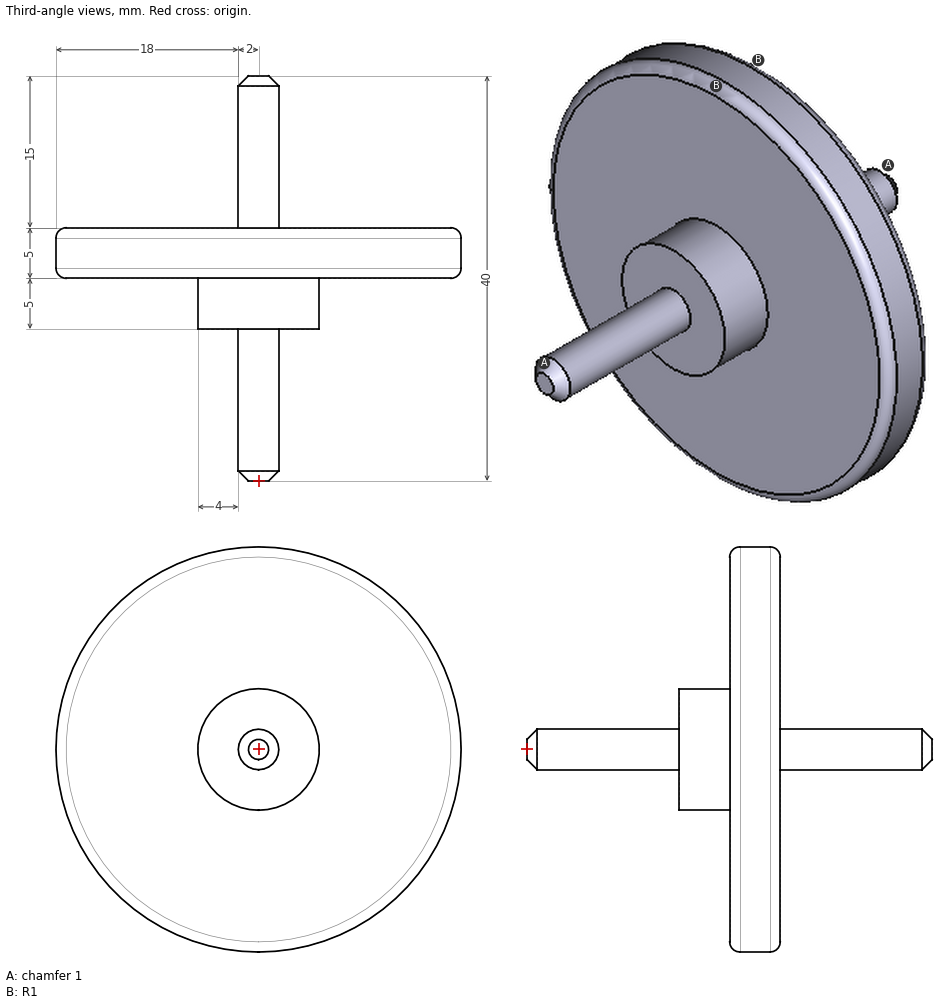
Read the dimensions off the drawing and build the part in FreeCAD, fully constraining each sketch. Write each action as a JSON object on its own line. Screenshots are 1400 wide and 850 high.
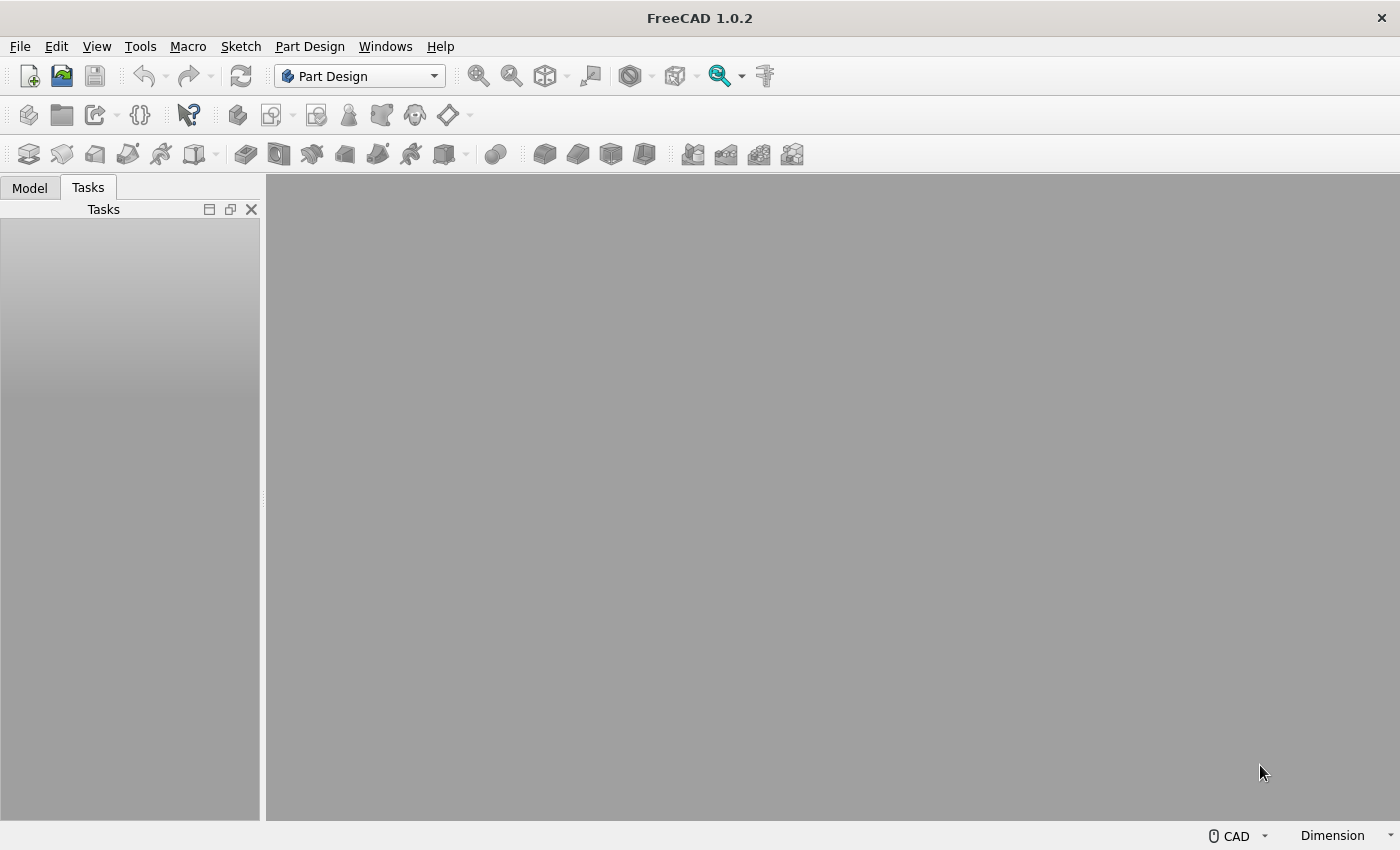
{"action": "key", "text": "ctrl+n"}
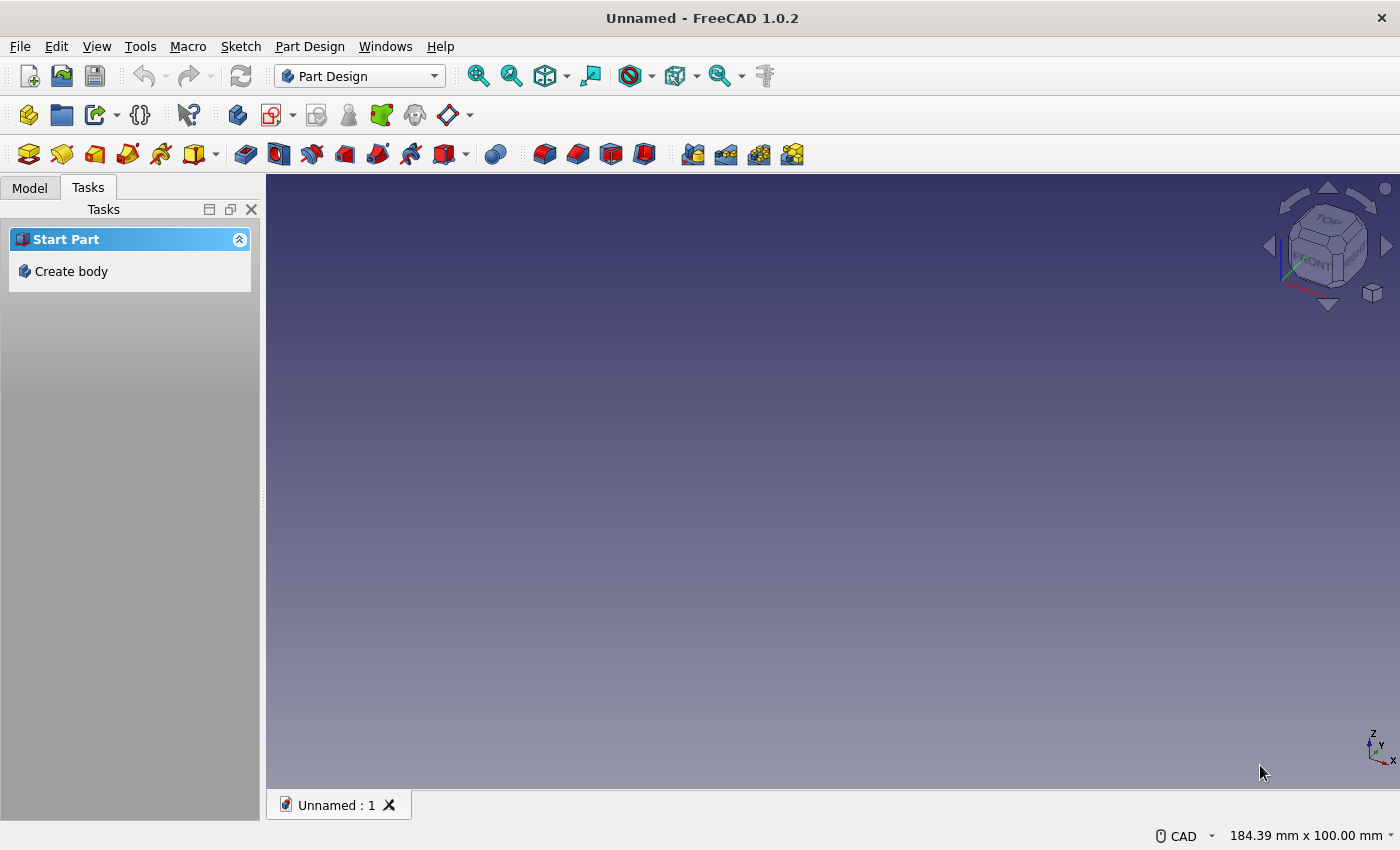
{"action": "left_click", "coordinate": [270, 116]}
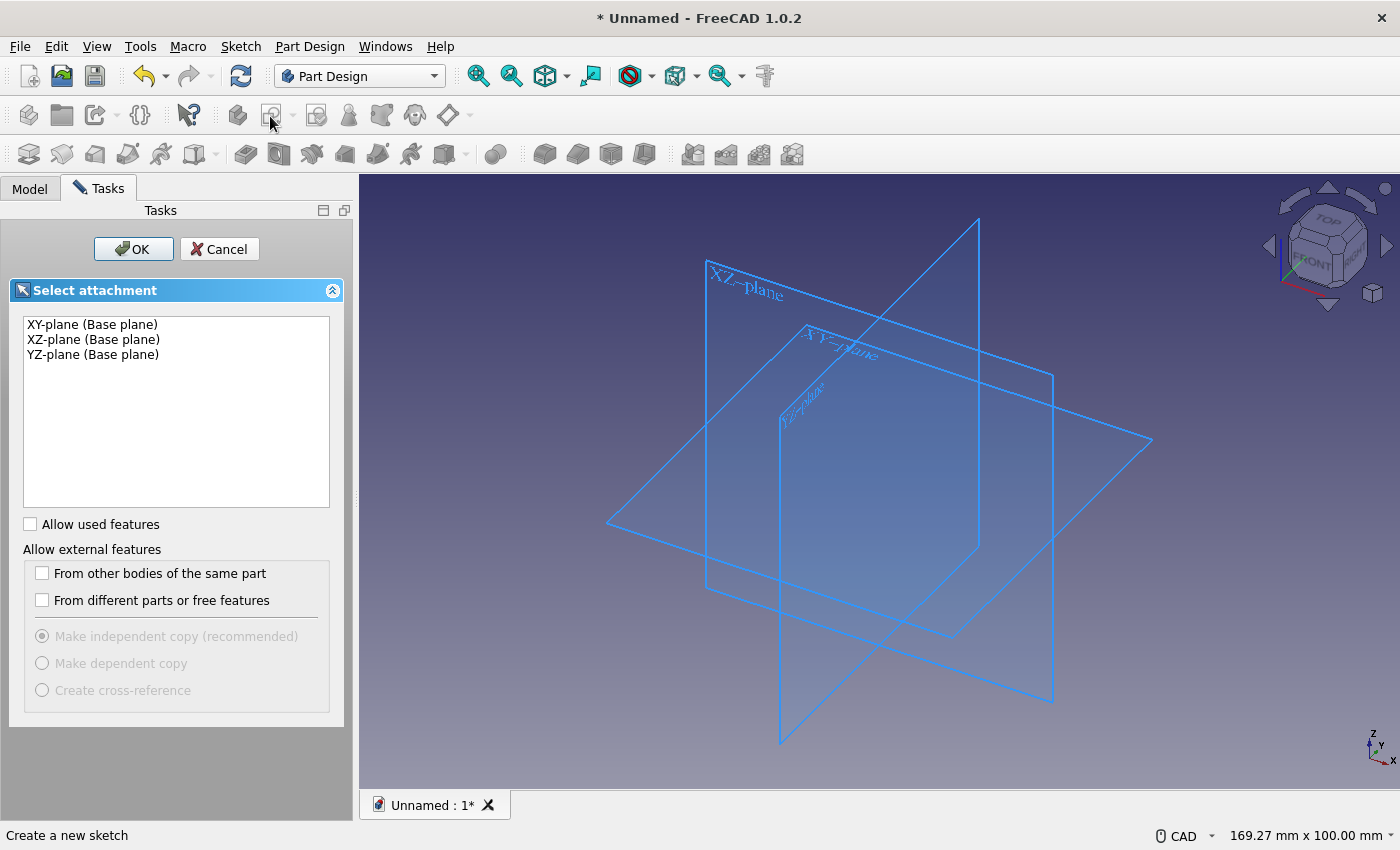
{"action": "left_click", "coordinate": [84, 324]}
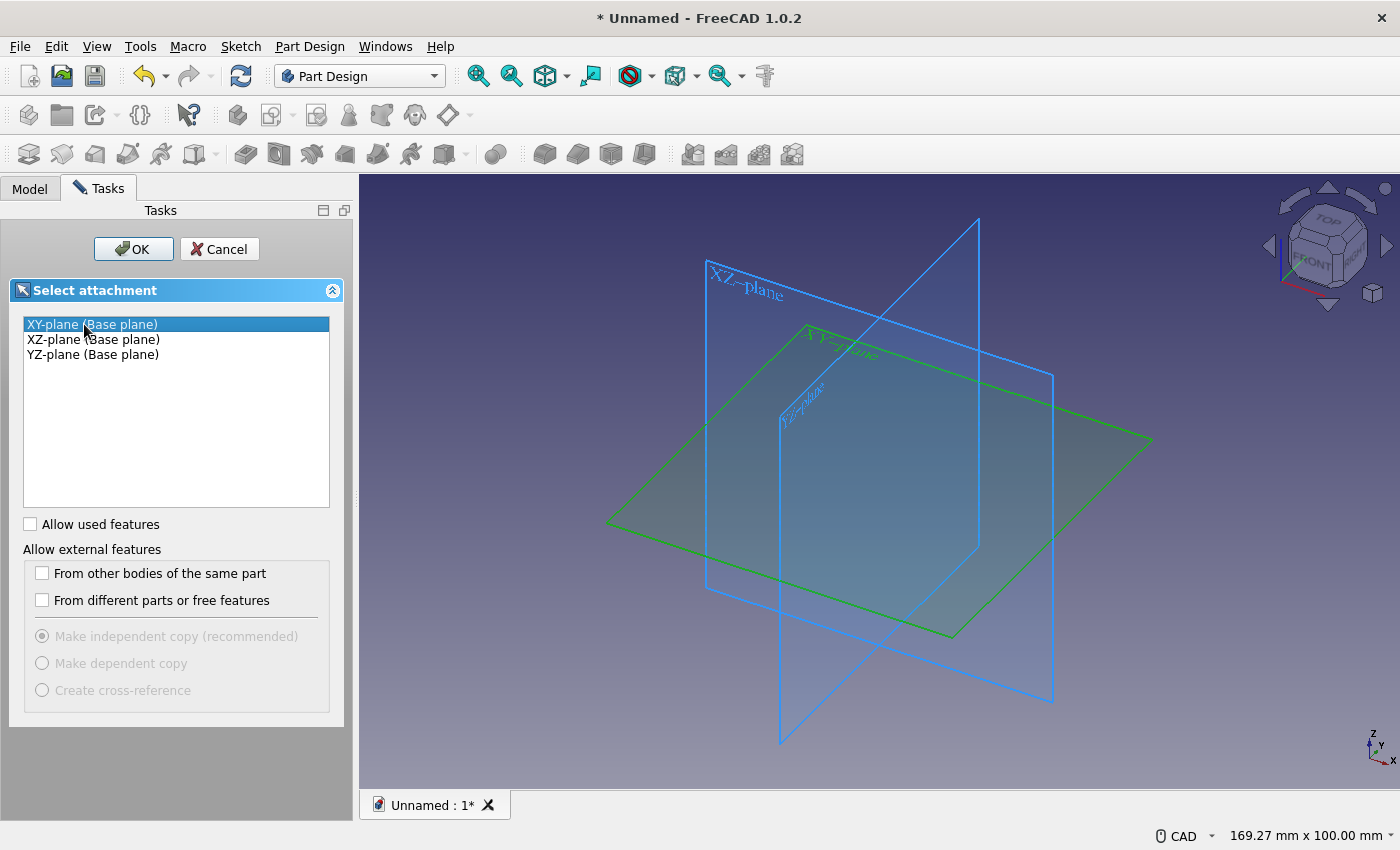
{"action": "left_click", "coordinate": [134, 249]}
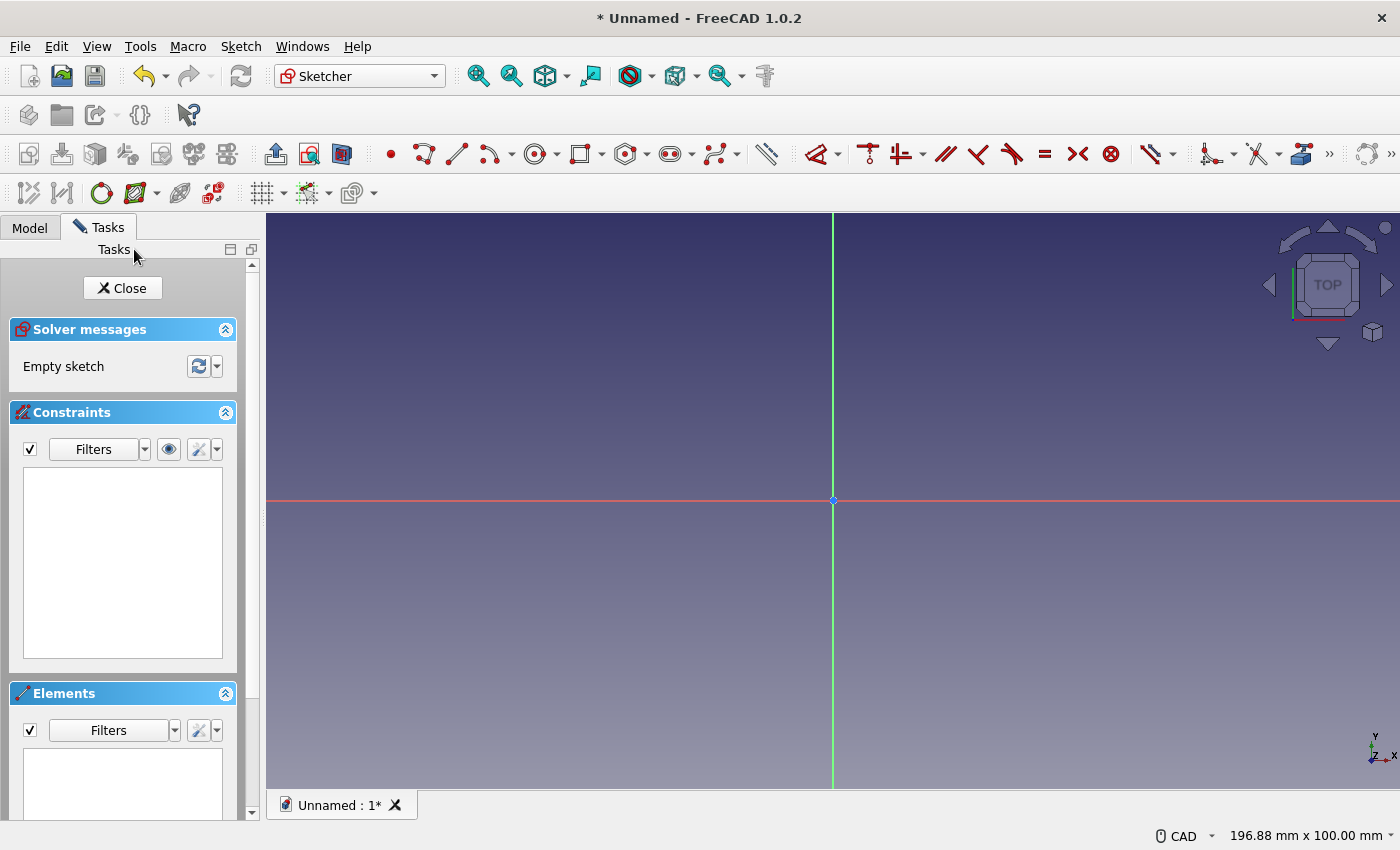
{"action": "scroll", "coordinate": [798, 241], "scroll_direction": "up", "scroll_amount": 2}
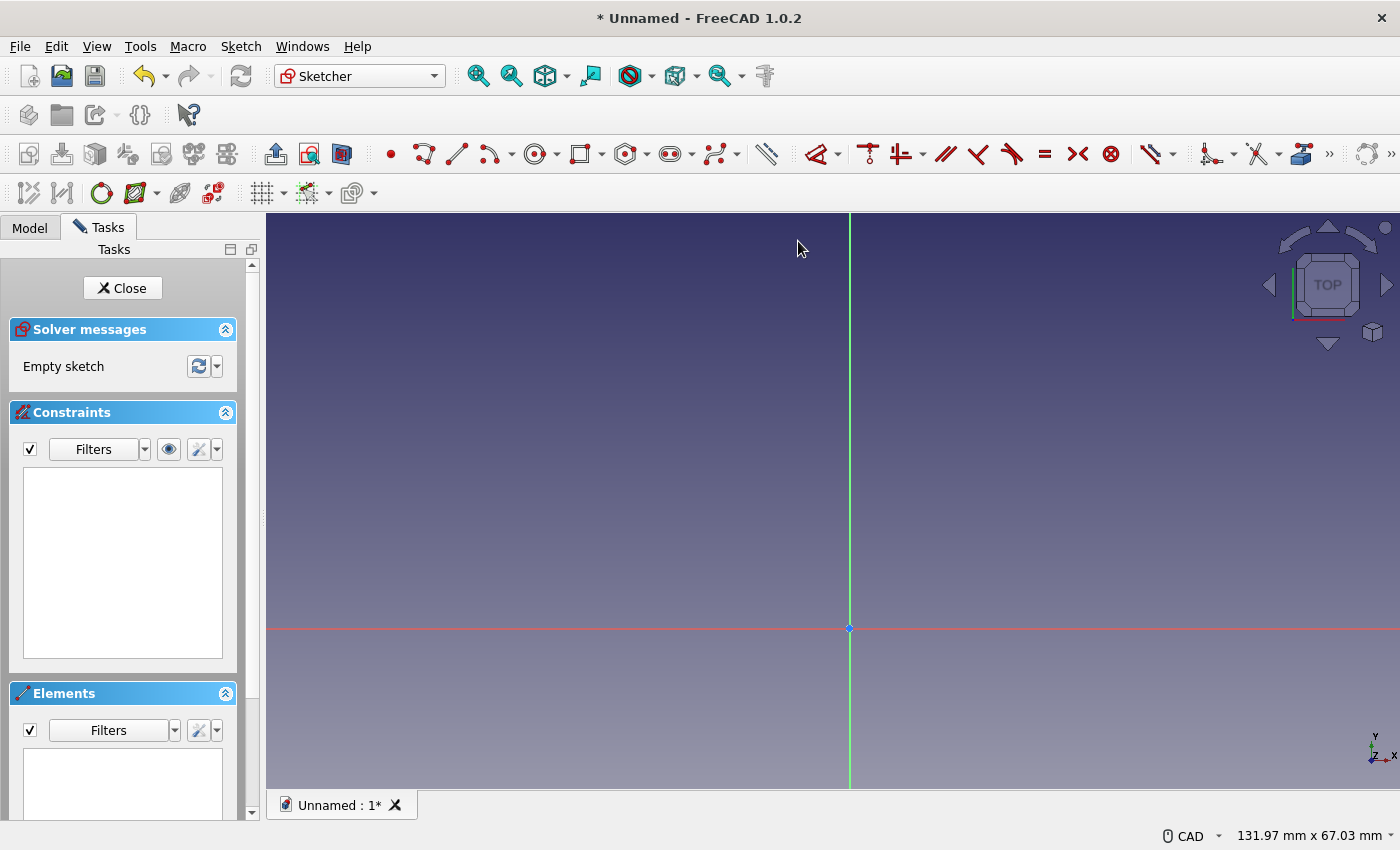
{"action": "left_click", "coordinate": [424, 154]}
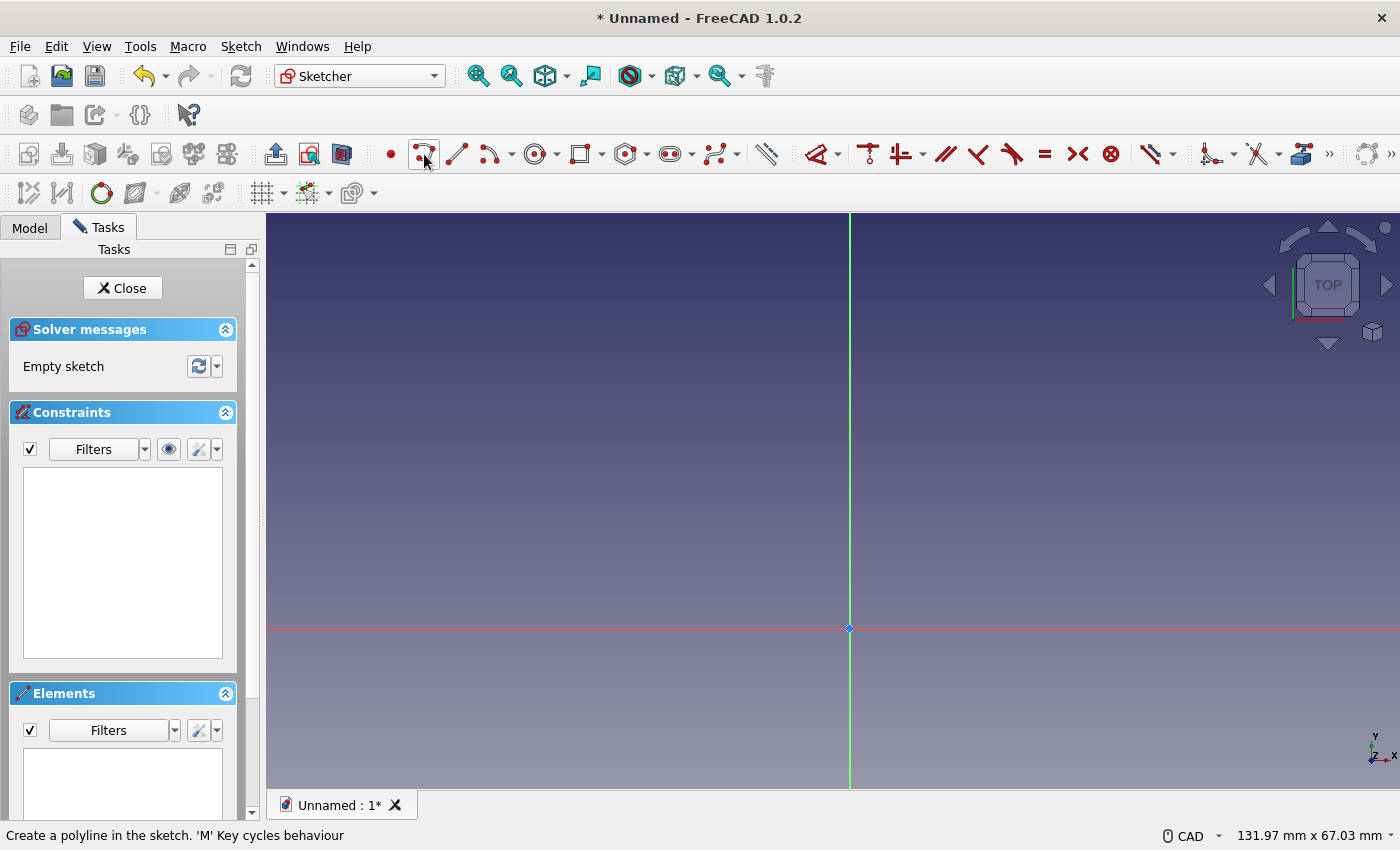
{"action": "left_click", "coordinate": [850, 629]}
{"action": "left_click", "coordinate": [841, 285]}
{"action": "left_click", "coordinate": [833, 285]}
{"action": "left_click", "coordinate": [833, 414]}
{"action": "left_click", "coordinate": [678, 414]}
{"action": "left_click", "coordinate": [678, 457]}
{"action": "left_click", "coordinate": [798, 457]}
{"action": "left_click", "coordinate": [798, 500]}
{"action": "left_click", "coordinate": [833, 500]}
{"action": "left_click", "coordinate": [833, 620]}
{"action": "left_click", "coordinate": [850, 629]}
{"action": "key", "text": "Escape"}
{"action": "key", "text": "Escape"}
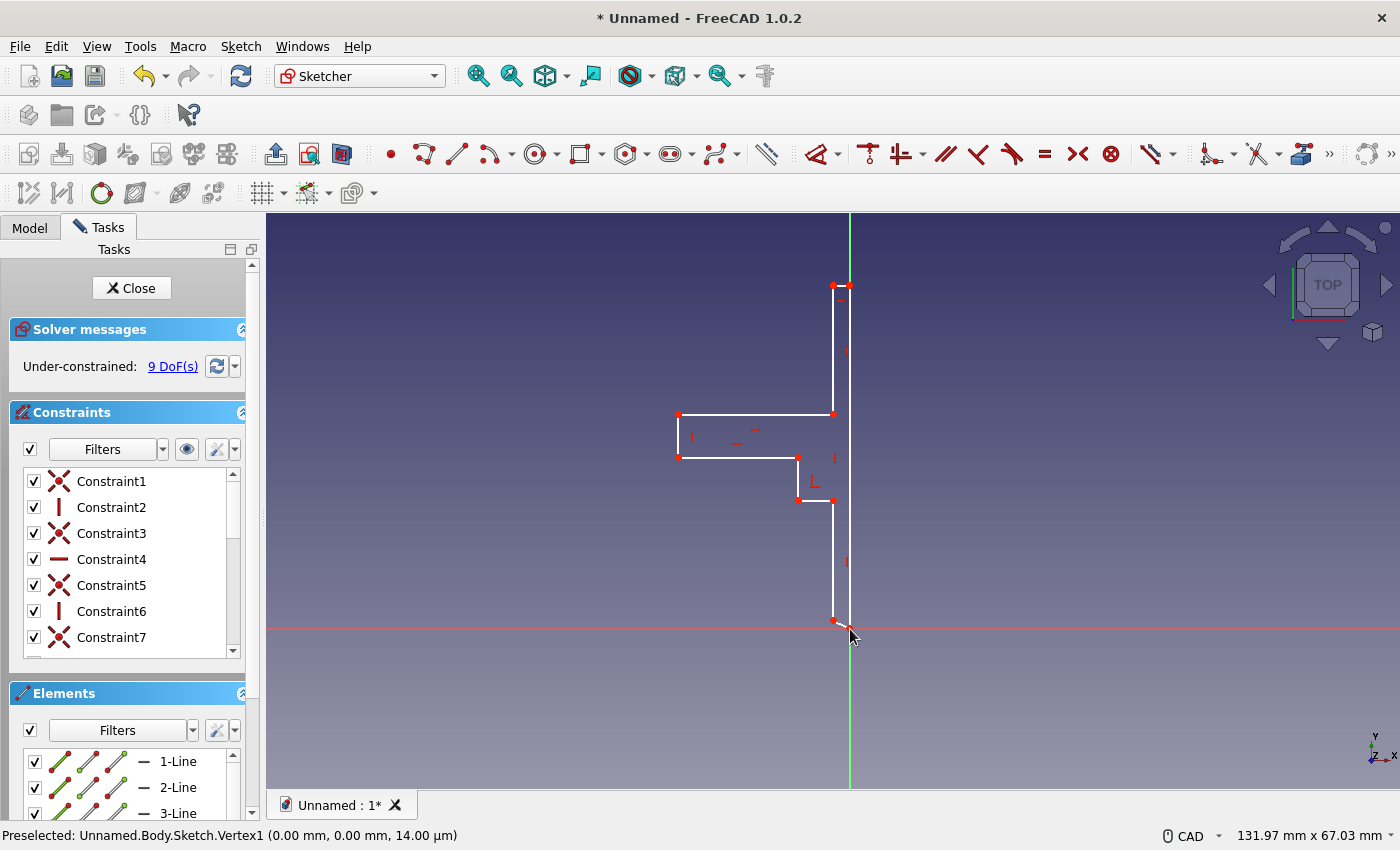
{"action": "scroll", "coordinate": [841, 625], "scroll_direction": "up", "scroll_amount": 3}